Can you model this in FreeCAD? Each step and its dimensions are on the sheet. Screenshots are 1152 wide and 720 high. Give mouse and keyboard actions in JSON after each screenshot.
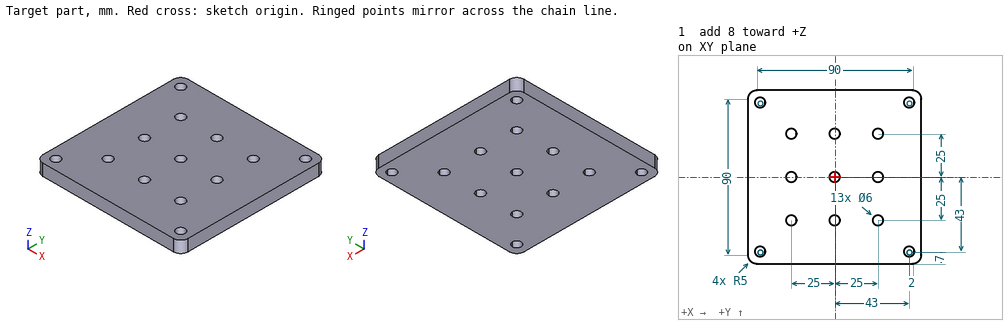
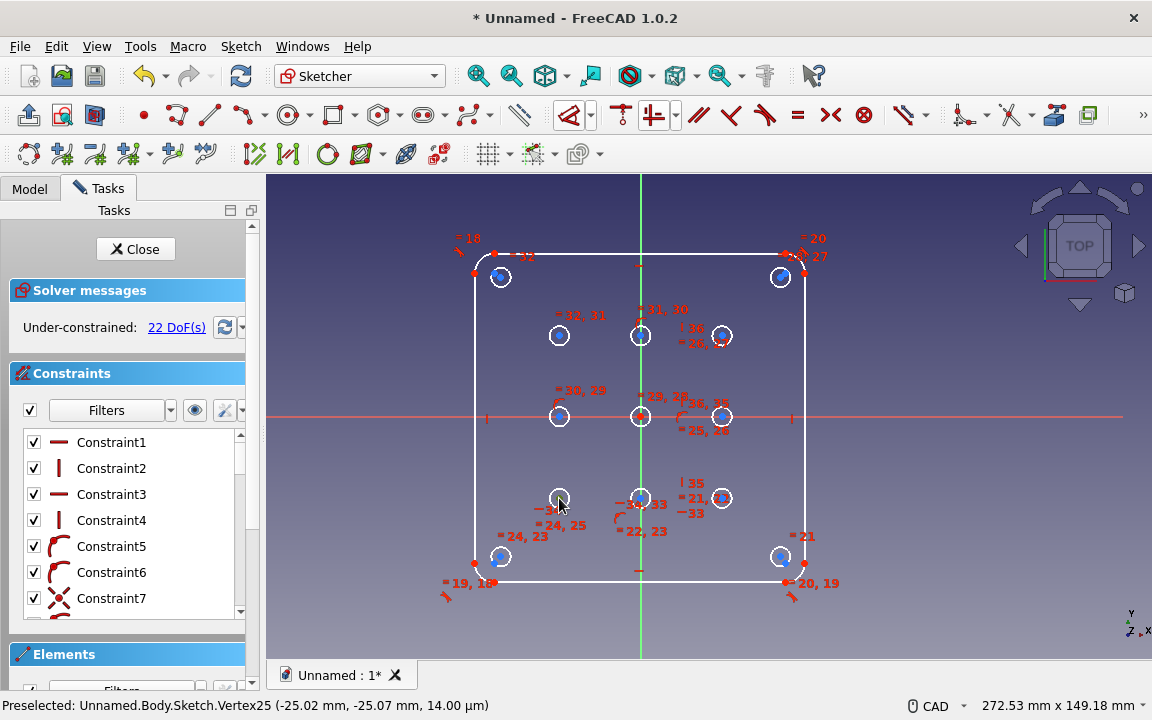
{"action": "left_click", "coordinate": [559, 417]}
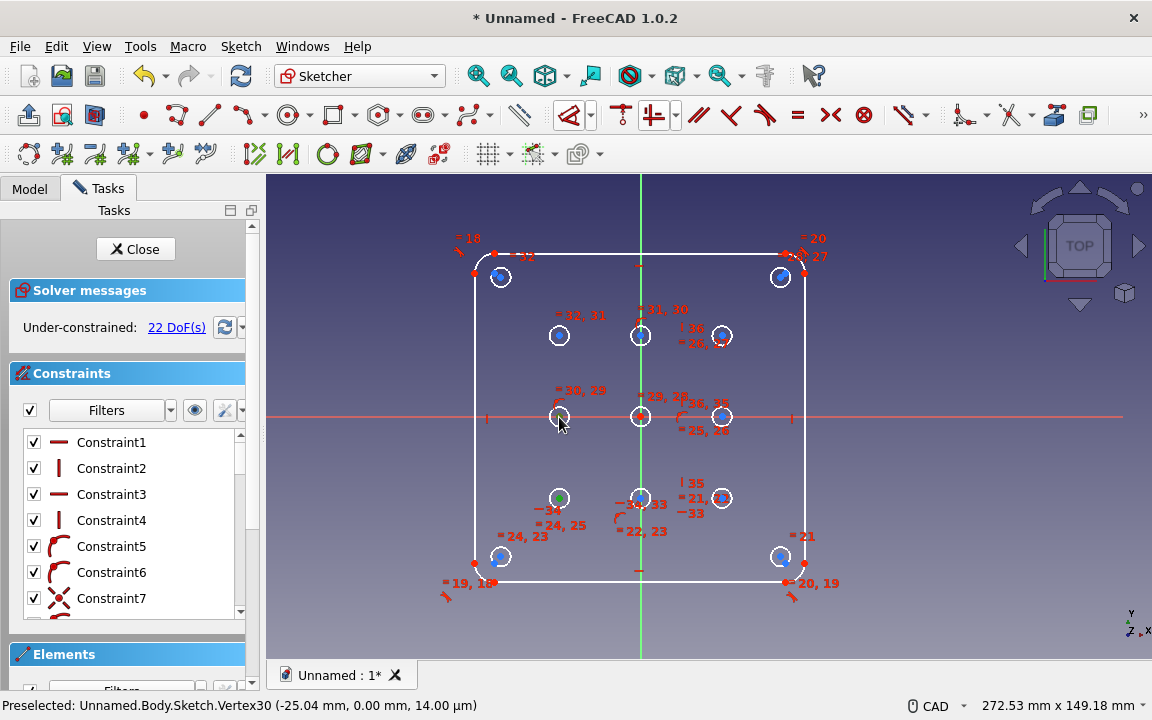
{"action": "key", "text": "v"}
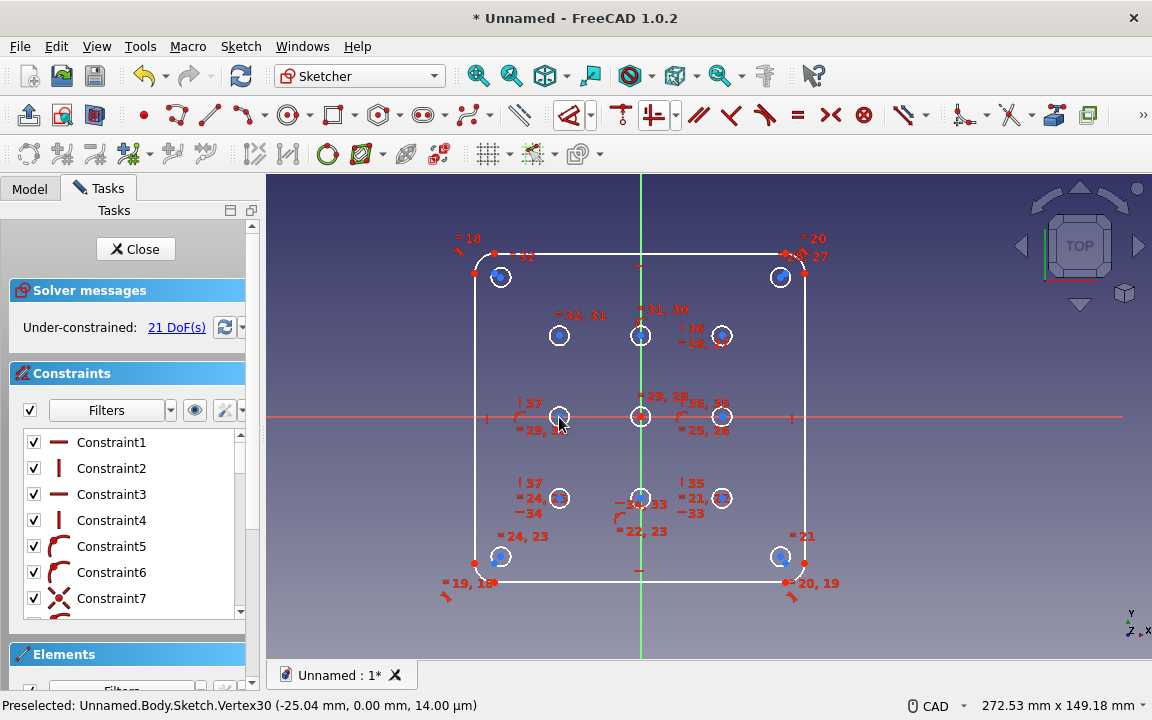
{"action": "scroll", "coordinate": [722, 336], "scroll_direction": "up", "scroll_amount": 4}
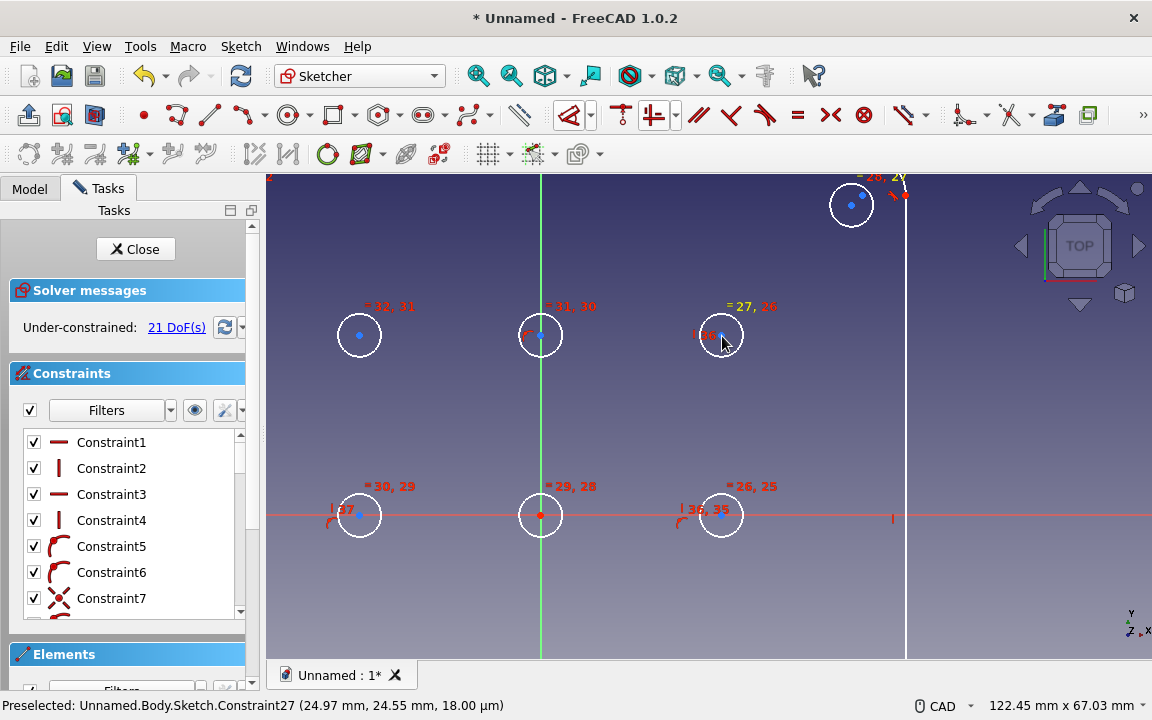
{"action": "left_click", "coordinate": [721, 335]}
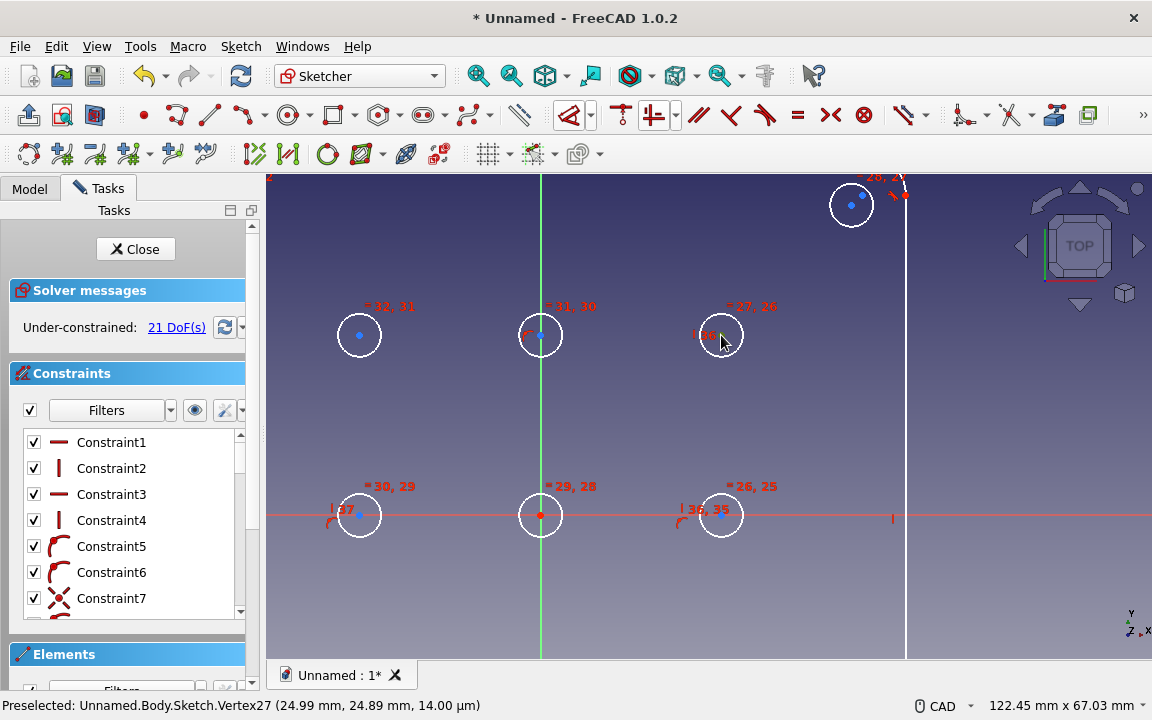
{"action": "left_click", "coordinate": [541, 335]}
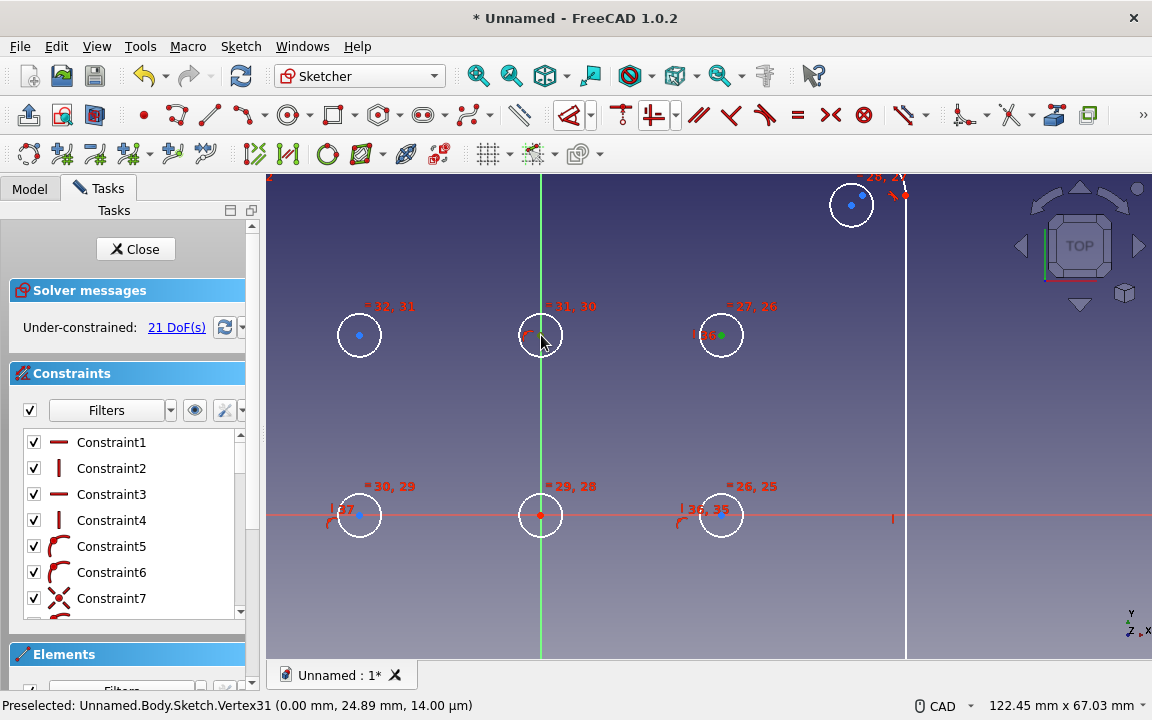
{"action": "left_click", "coordinate": [676, 116]}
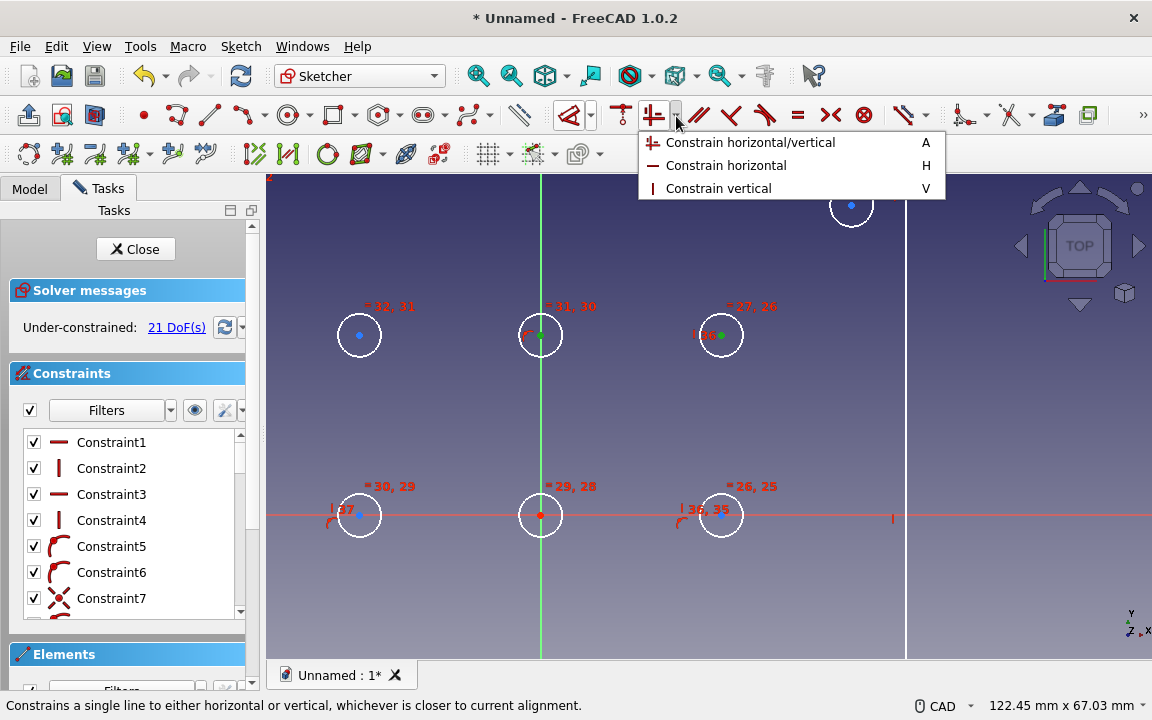
{"action": "left_click", "coordinate": [792, 166]}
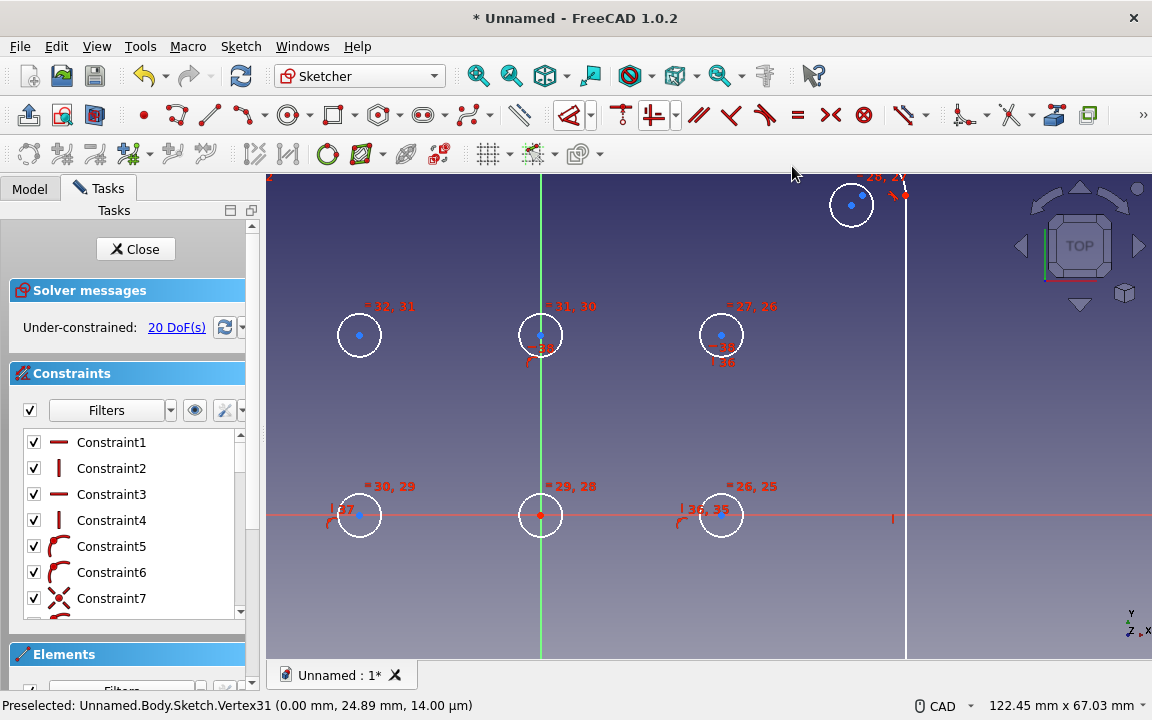
{"action": "left_click", "coordinate": [360, 515]}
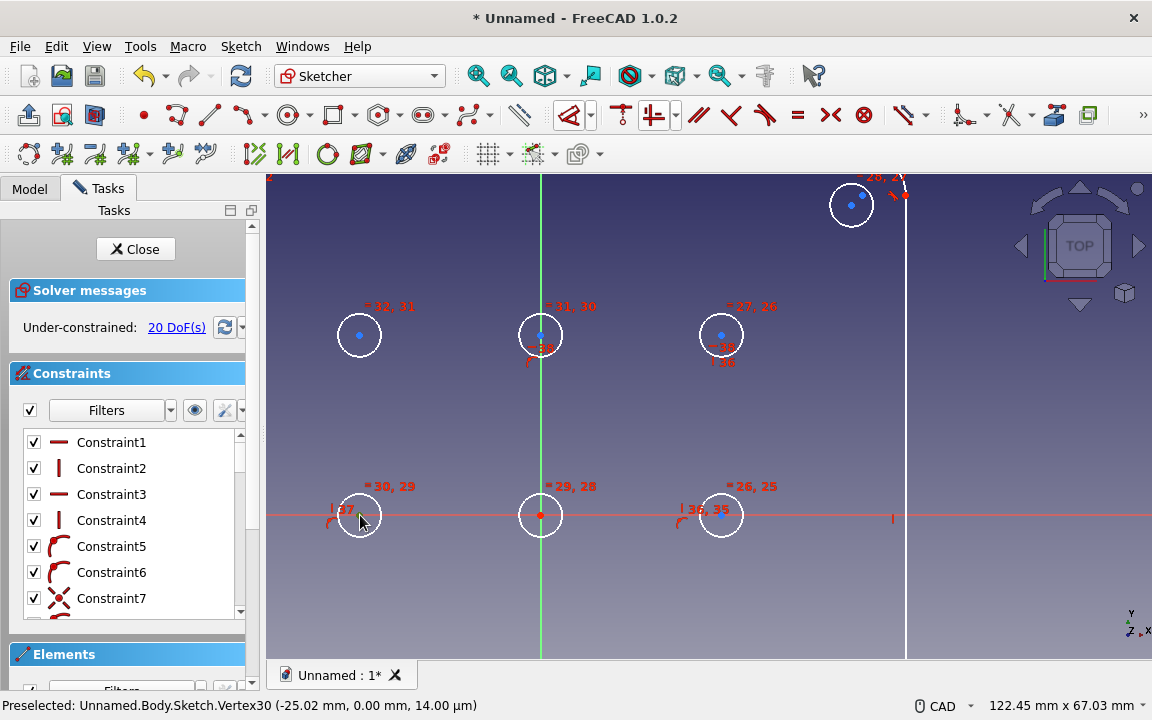
{"action": "left_click", "coordinate": [360, 335]}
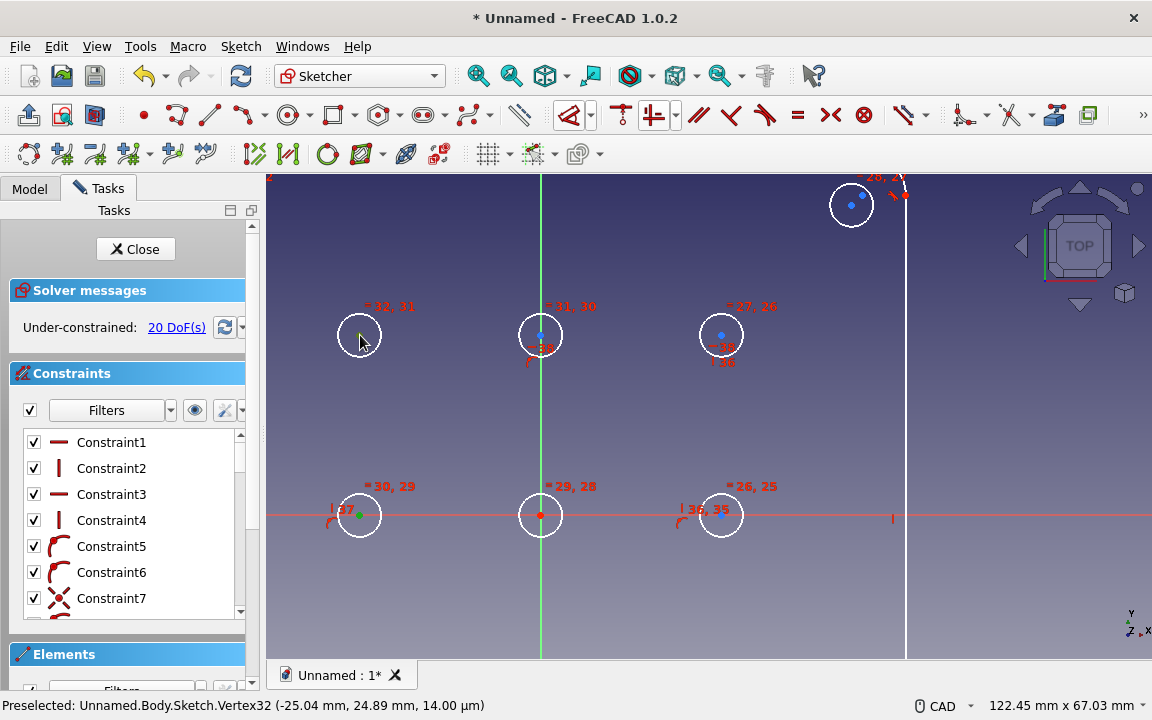
{"action": "key", "text": "v"}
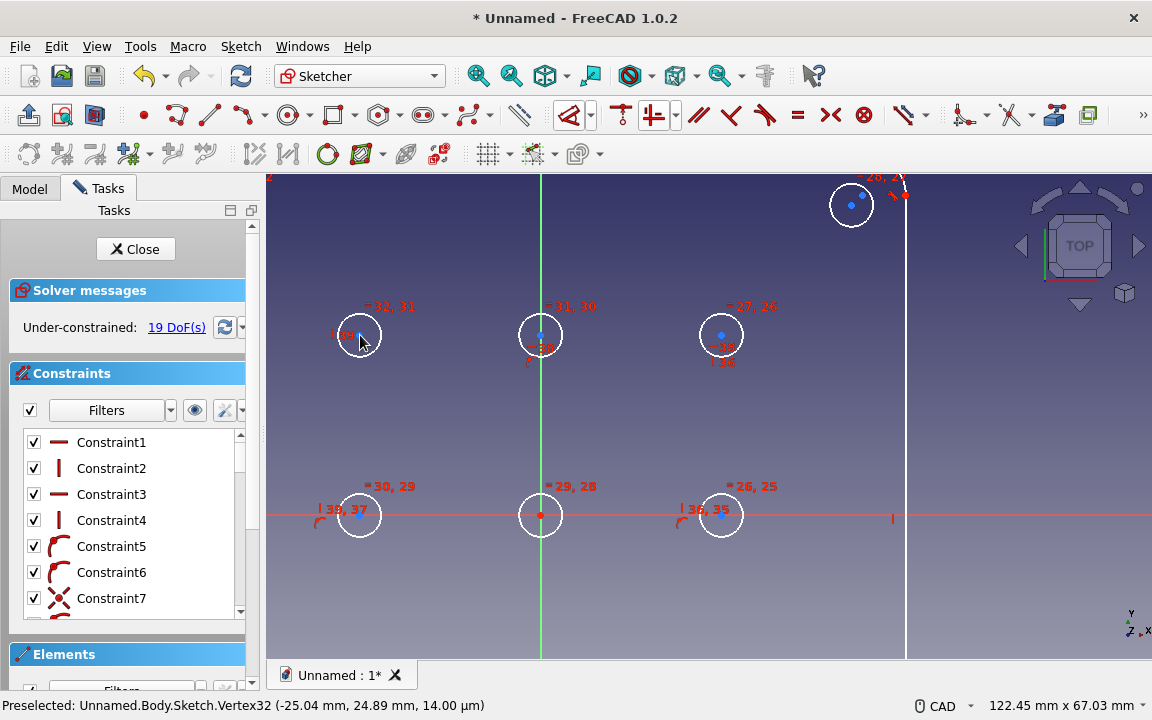
{"action": "left_click", "coordinate": [541, 335]}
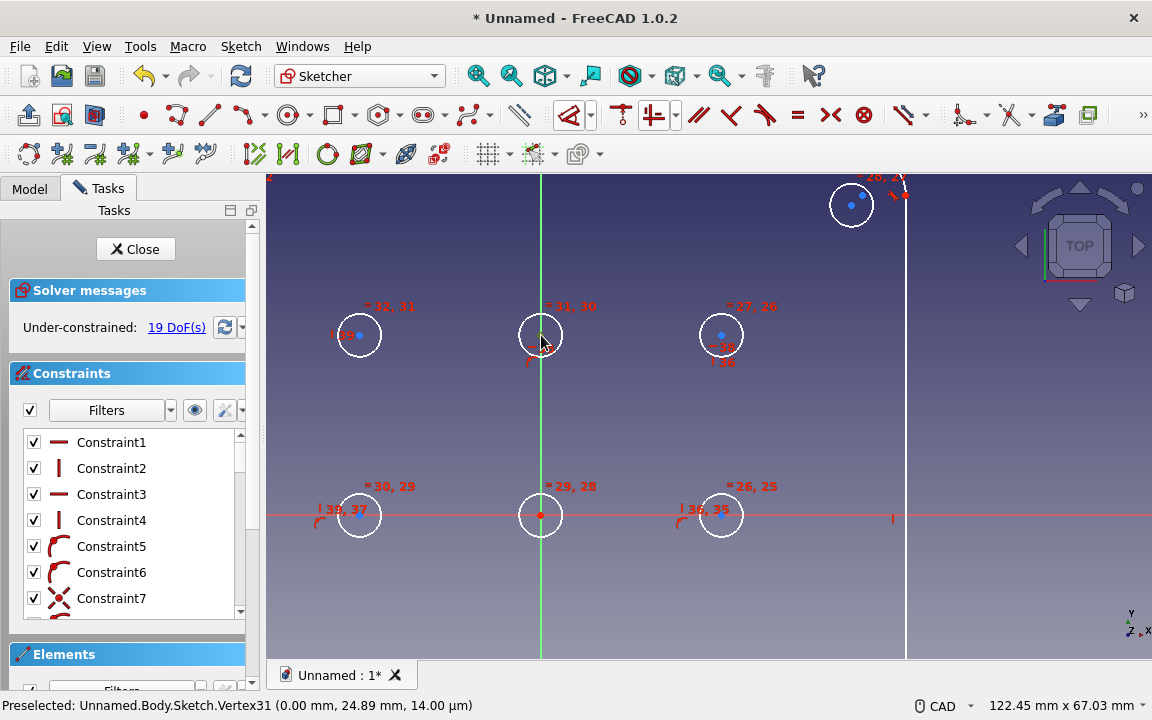
{"action": "left_click", "coordinate": [360, 335]}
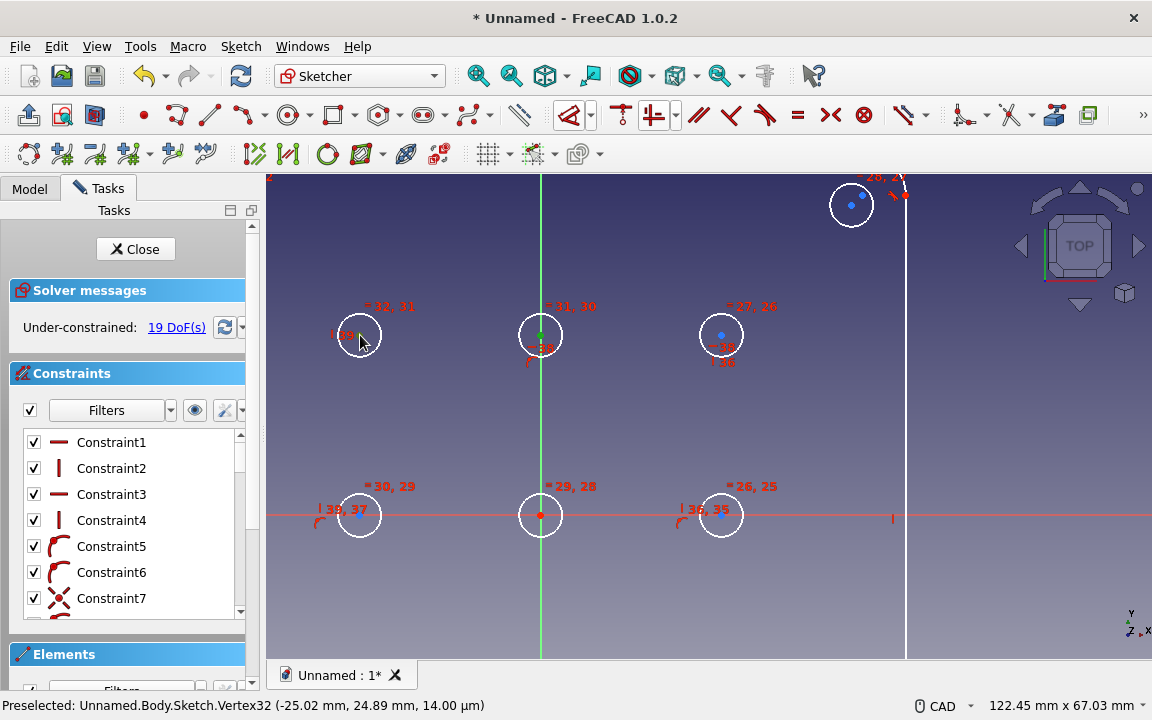
{"action": "key", "text": "h"}